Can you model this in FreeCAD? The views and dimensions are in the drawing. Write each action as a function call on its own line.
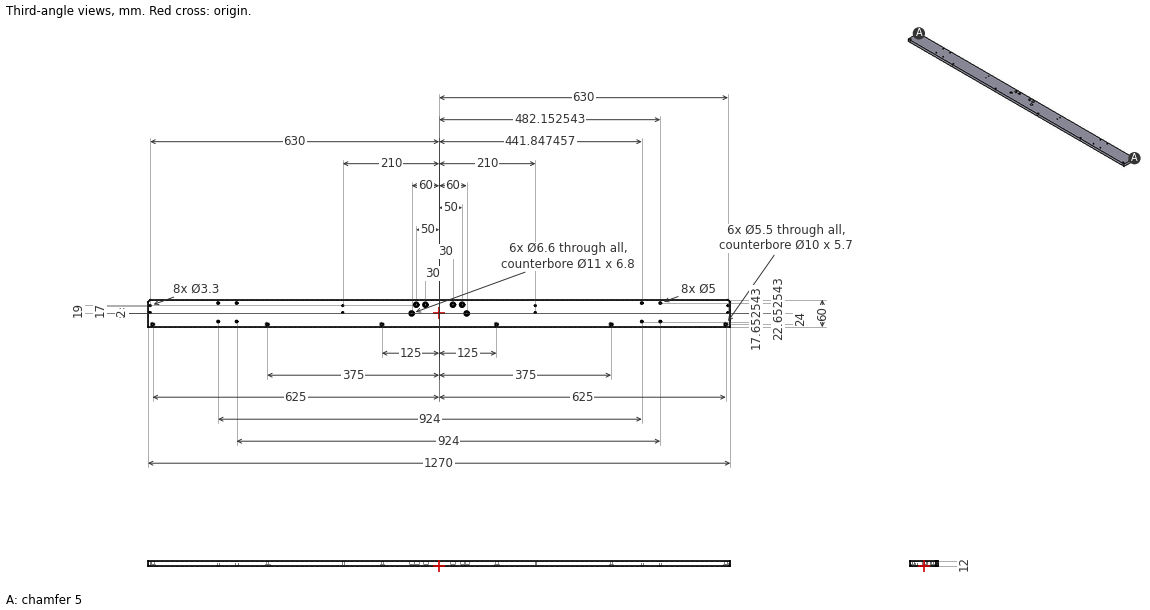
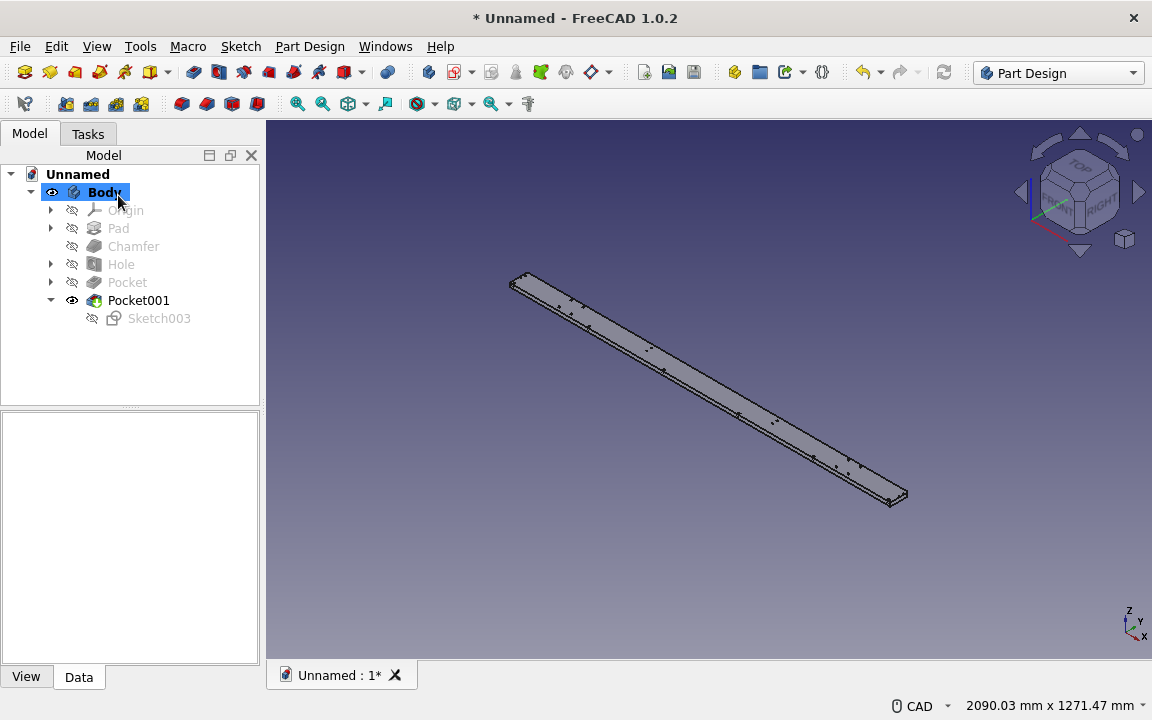
key(v)
key(f)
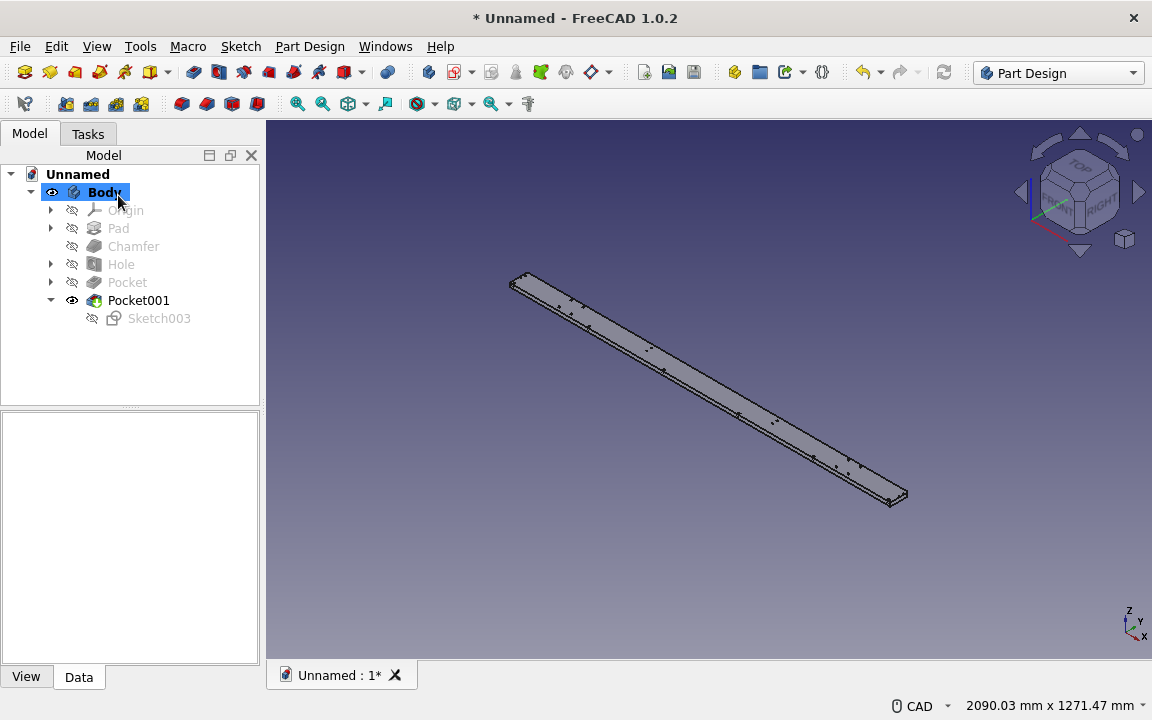
click(709, 386)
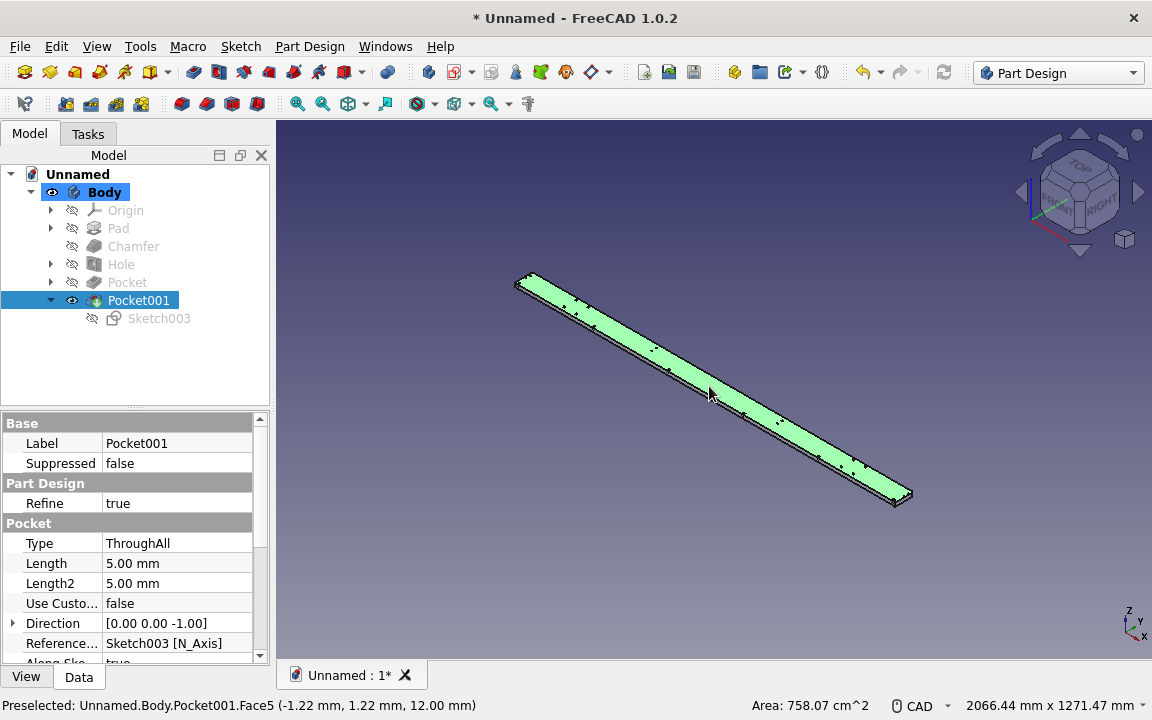
click(454, 72)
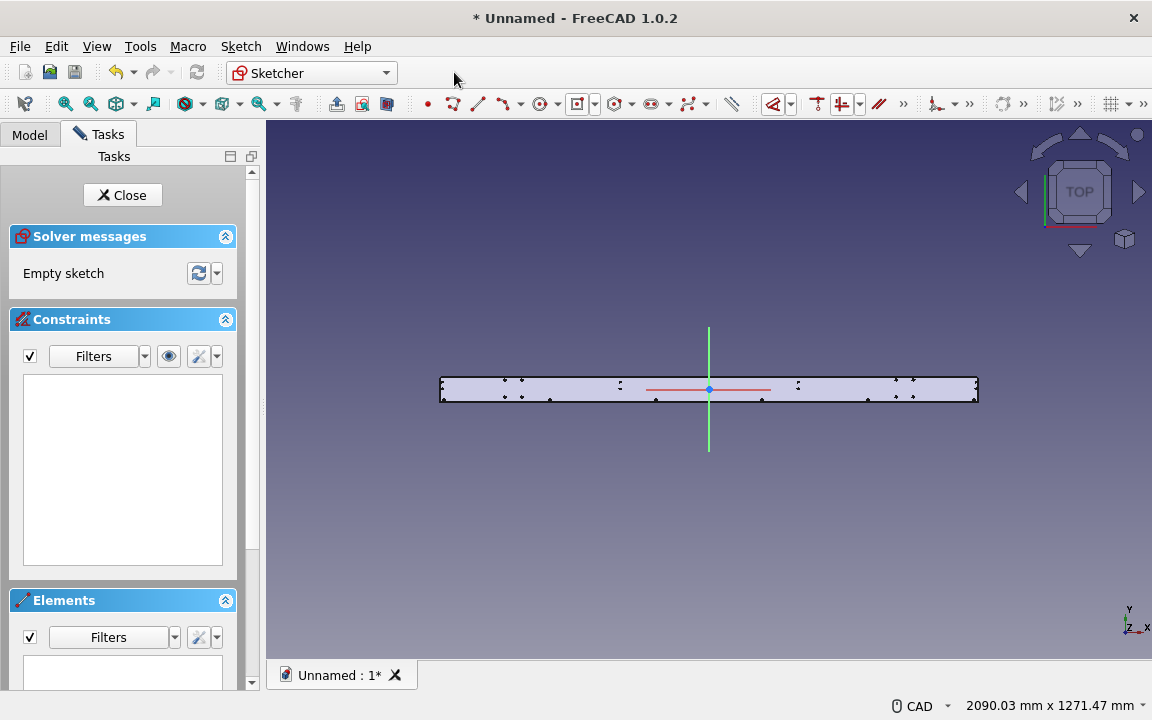
scroll(718, 385, up, 11)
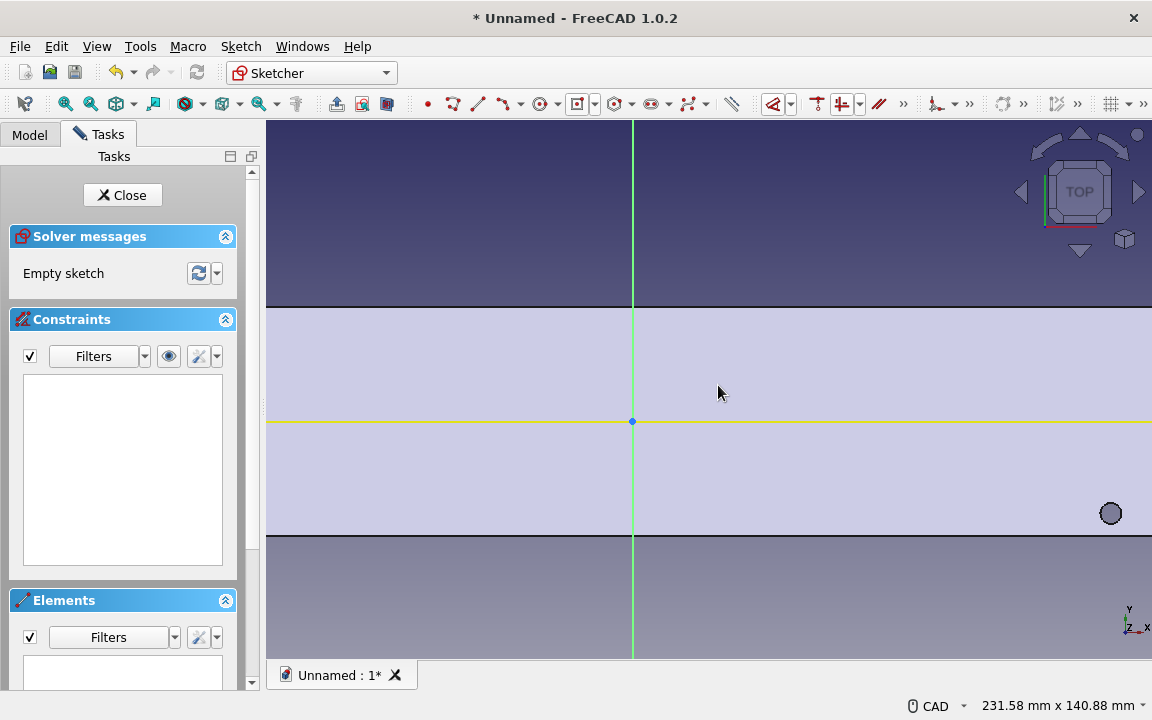
click(540, 104)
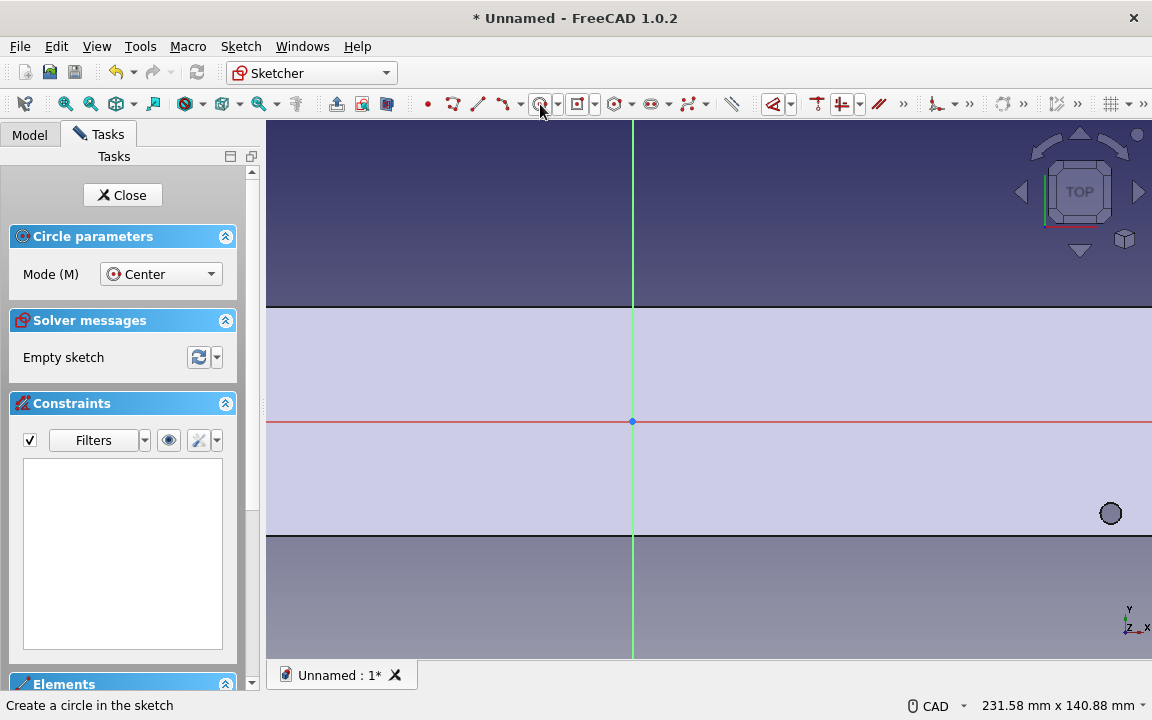
scroll(403, 422, up, 3)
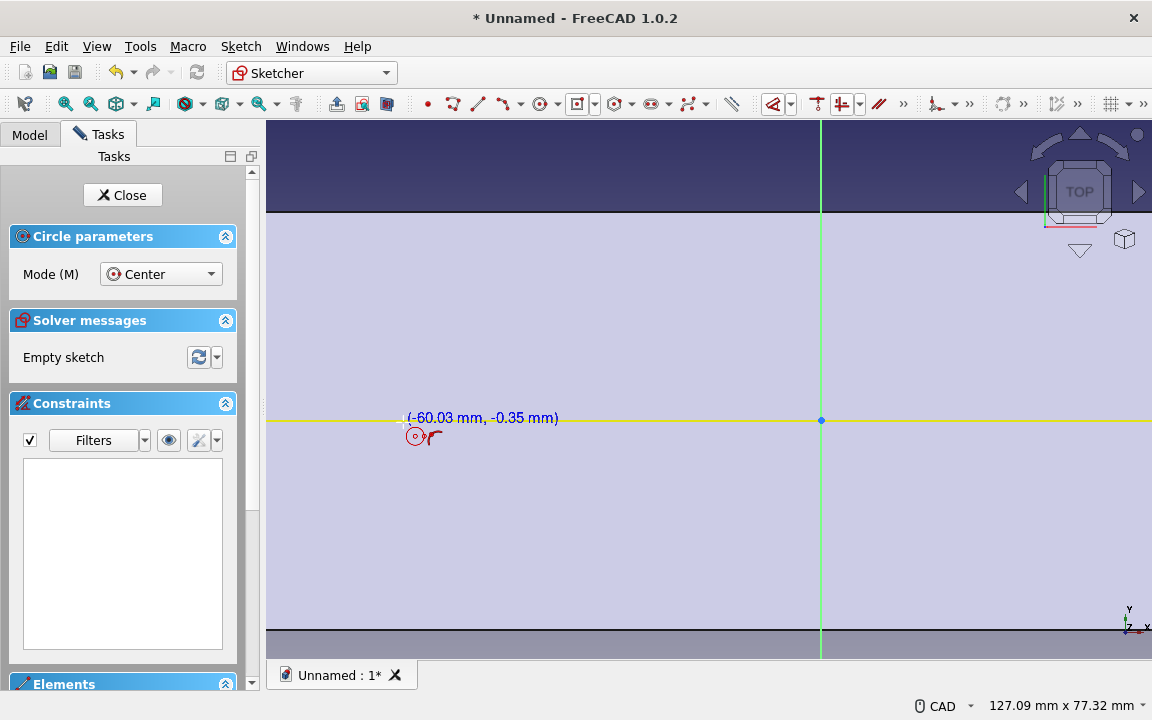
click(403, 421)
click(419, 405)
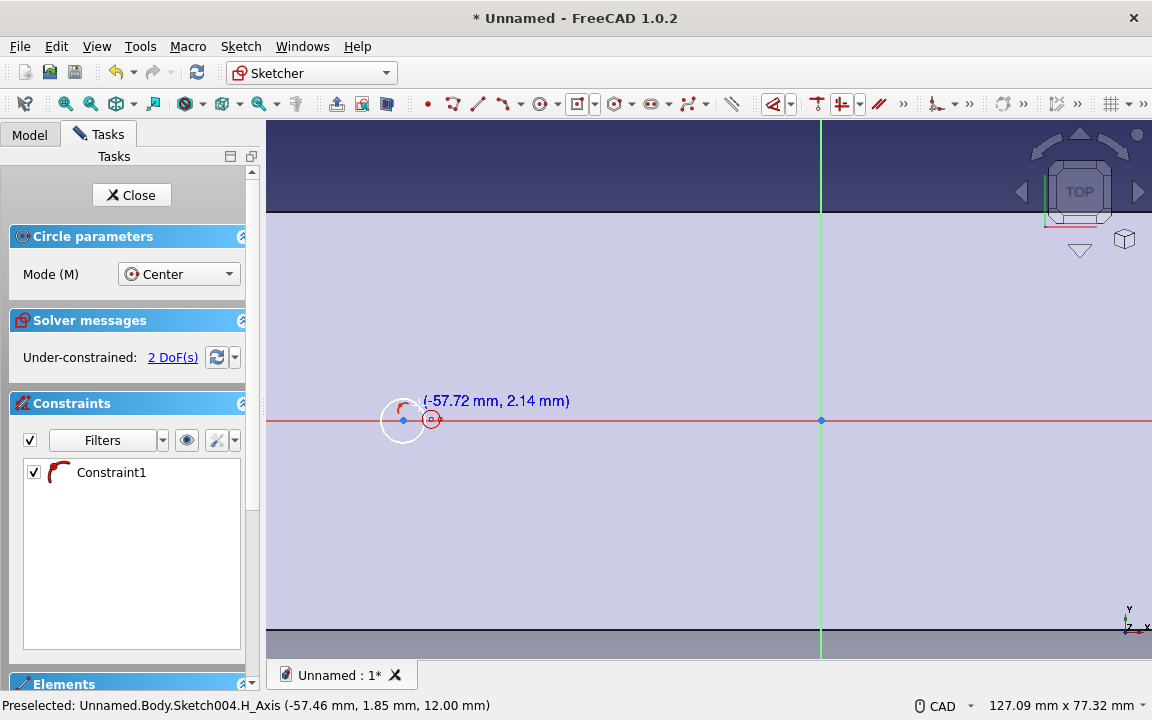
click(473, 288)
click(489, 272)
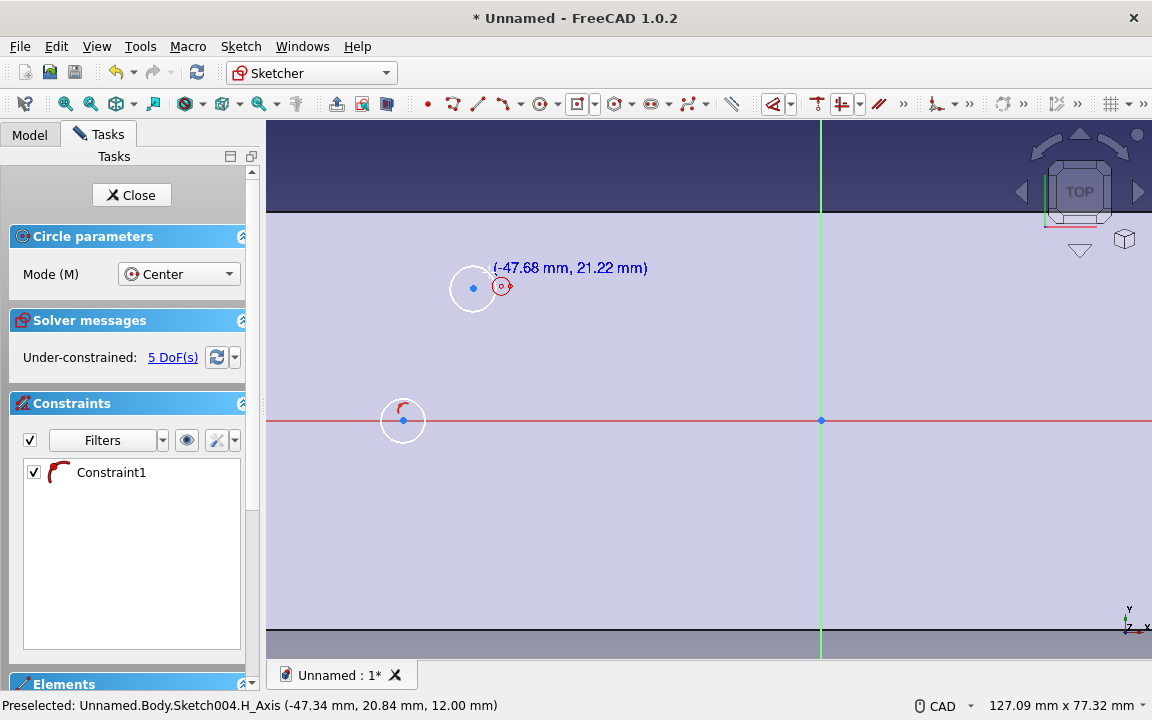
click(612, 288)
click(629, 272)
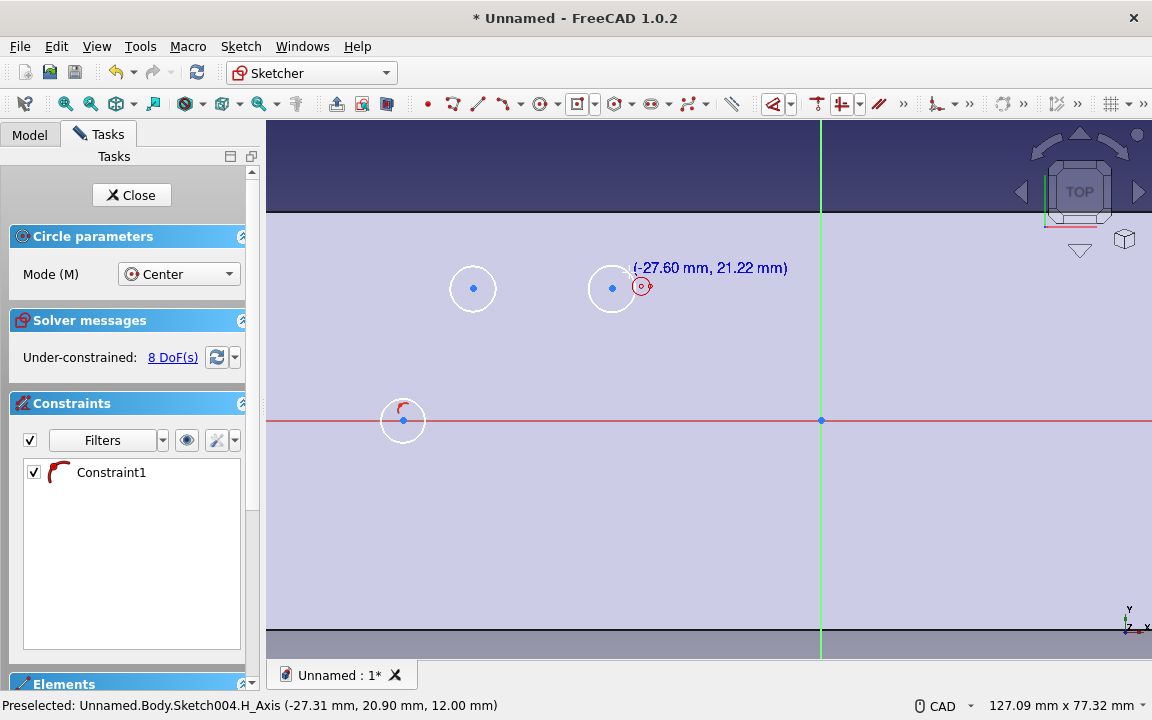
scroll(420, 432, down, 3)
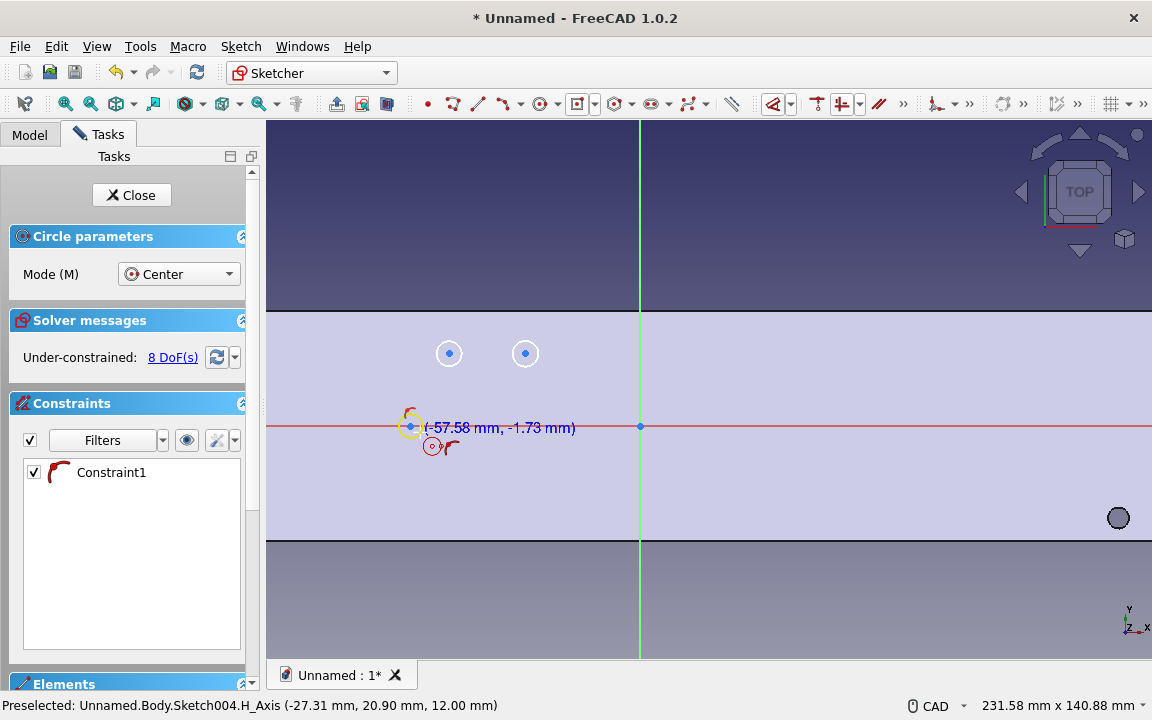
scroll(755, 353, up, 3)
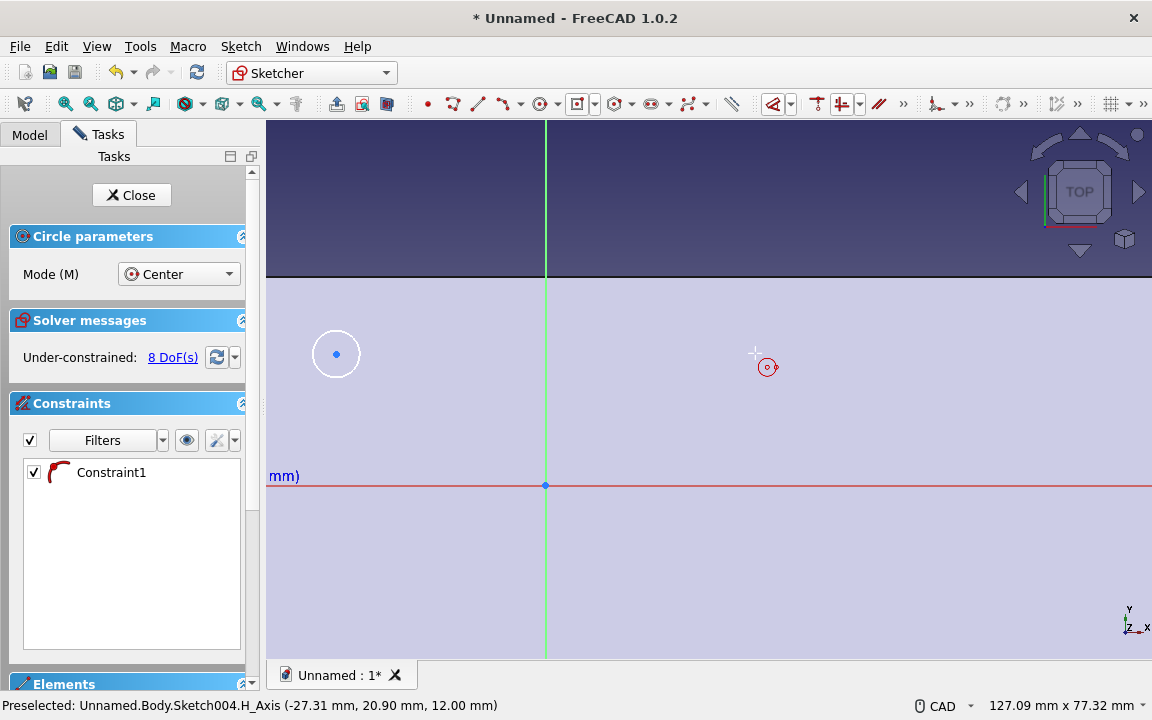
click(755, 354)
click(771, 337)